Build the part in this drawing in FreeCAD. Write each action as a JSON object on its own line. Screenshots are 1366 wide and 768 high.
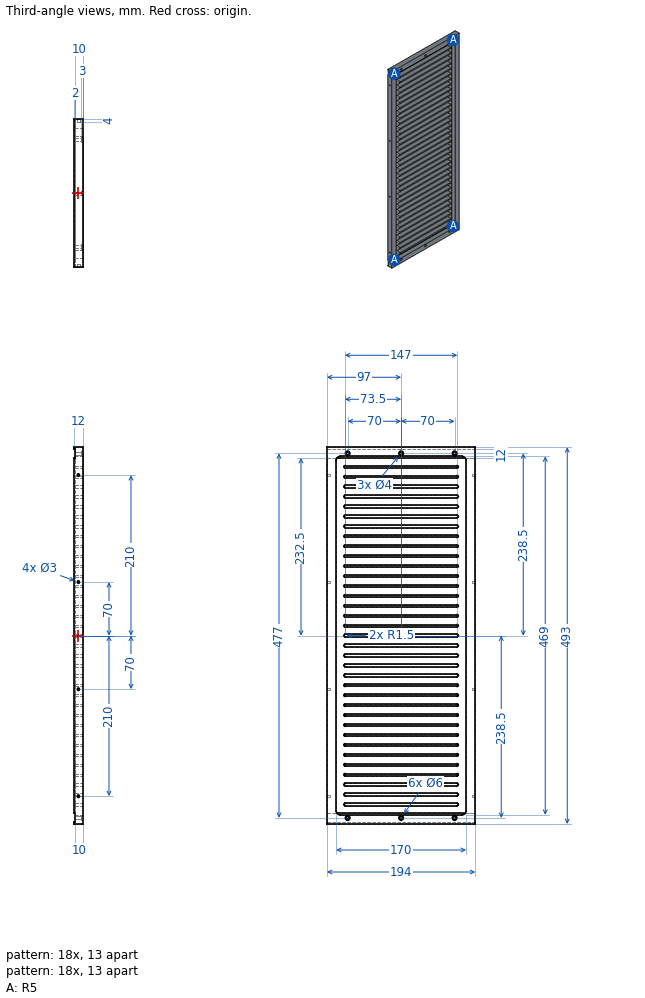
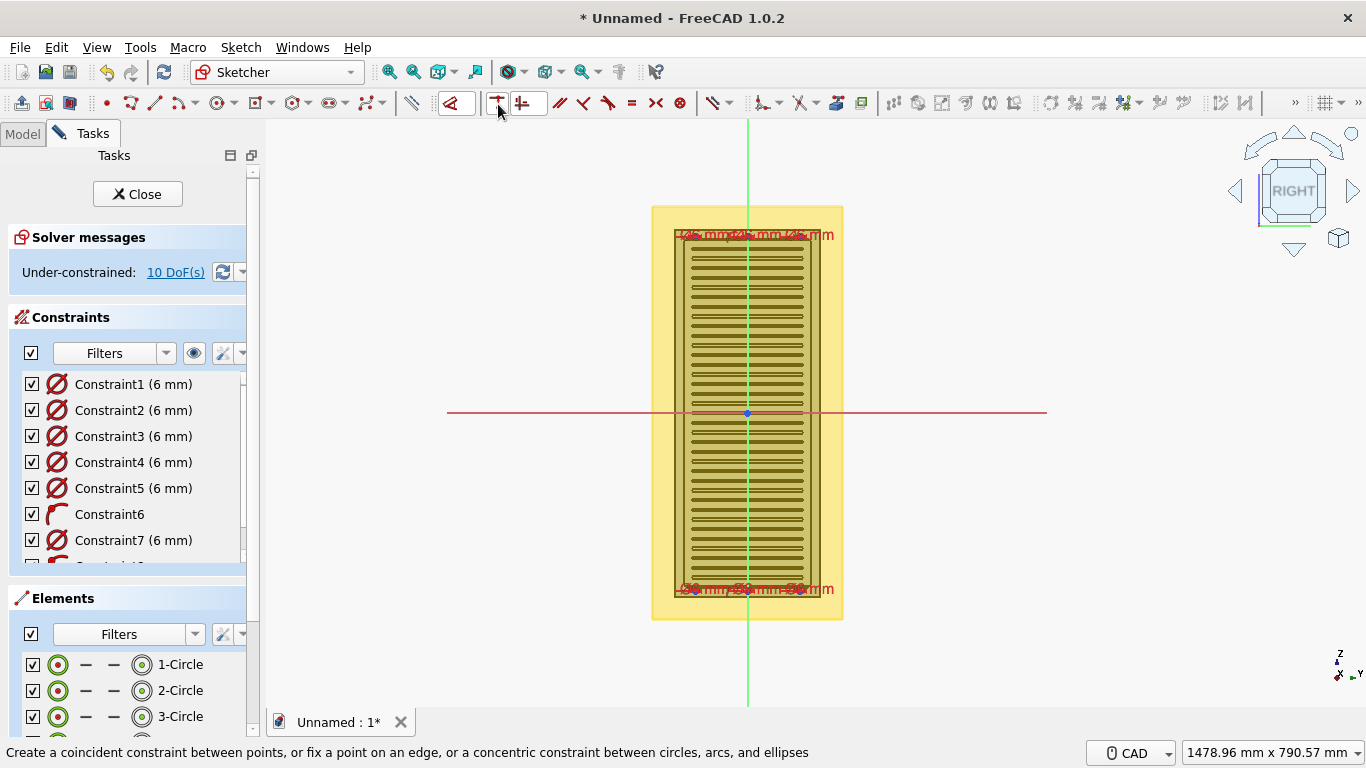
{"action": "left_click", "coordinate": [748, 591]}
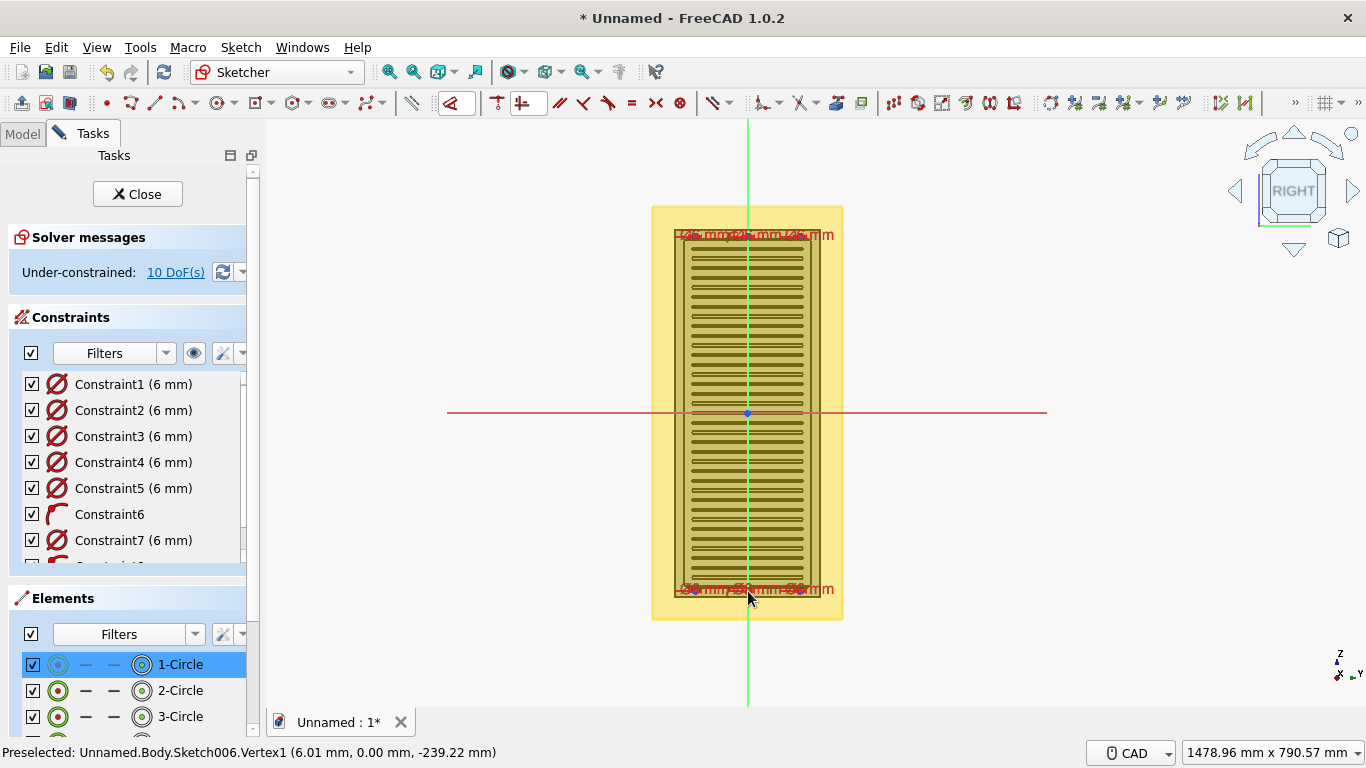
{"action": "left_click", "coordinate": [800, 591]}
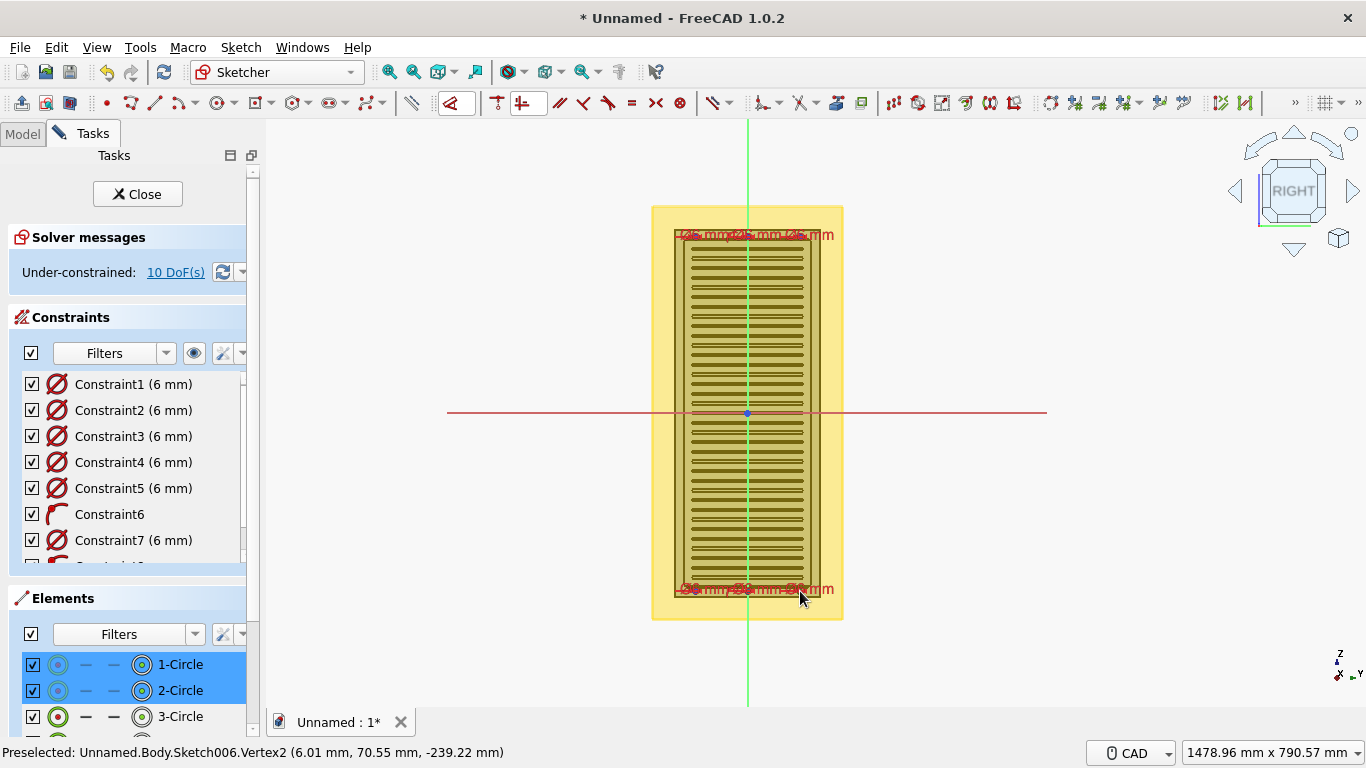
{"action": "key", "text": "h"}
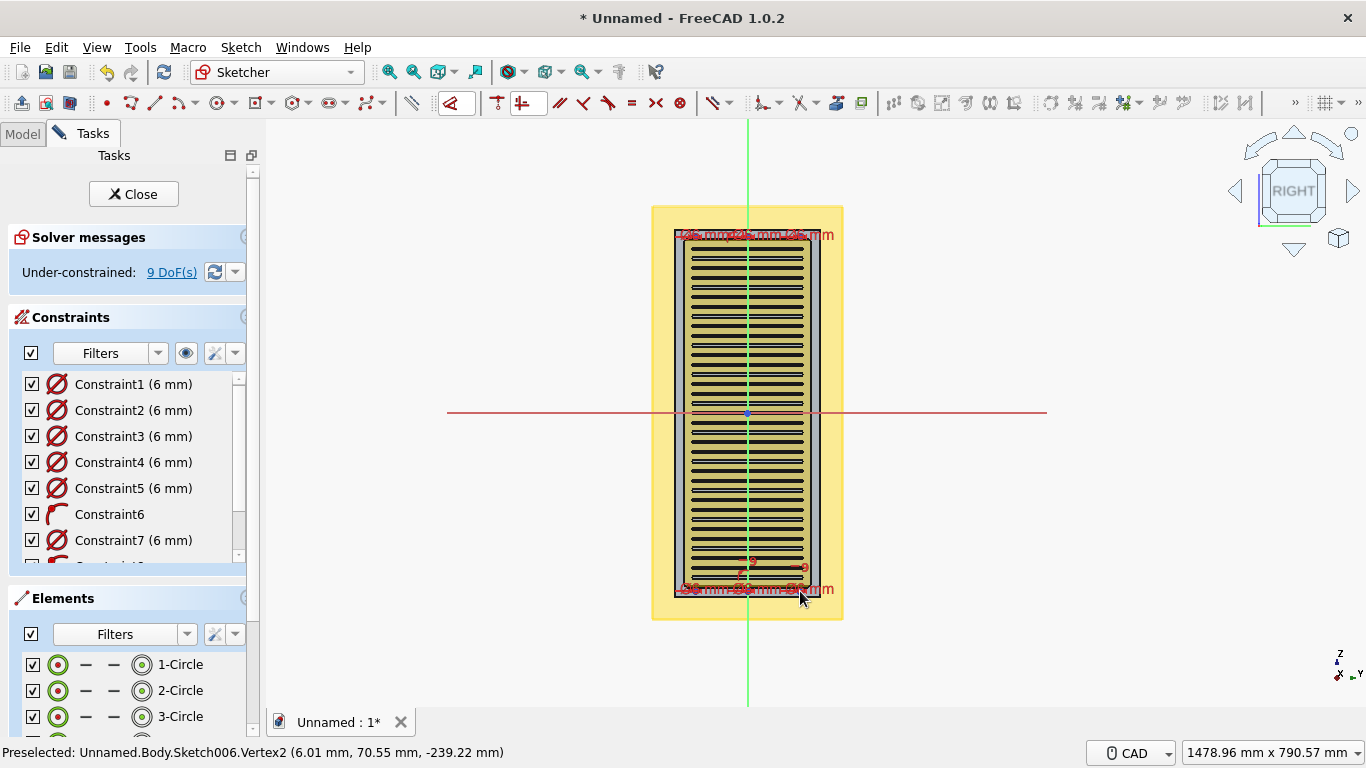
{"action": "left_click", "coordinate": [748, 591]}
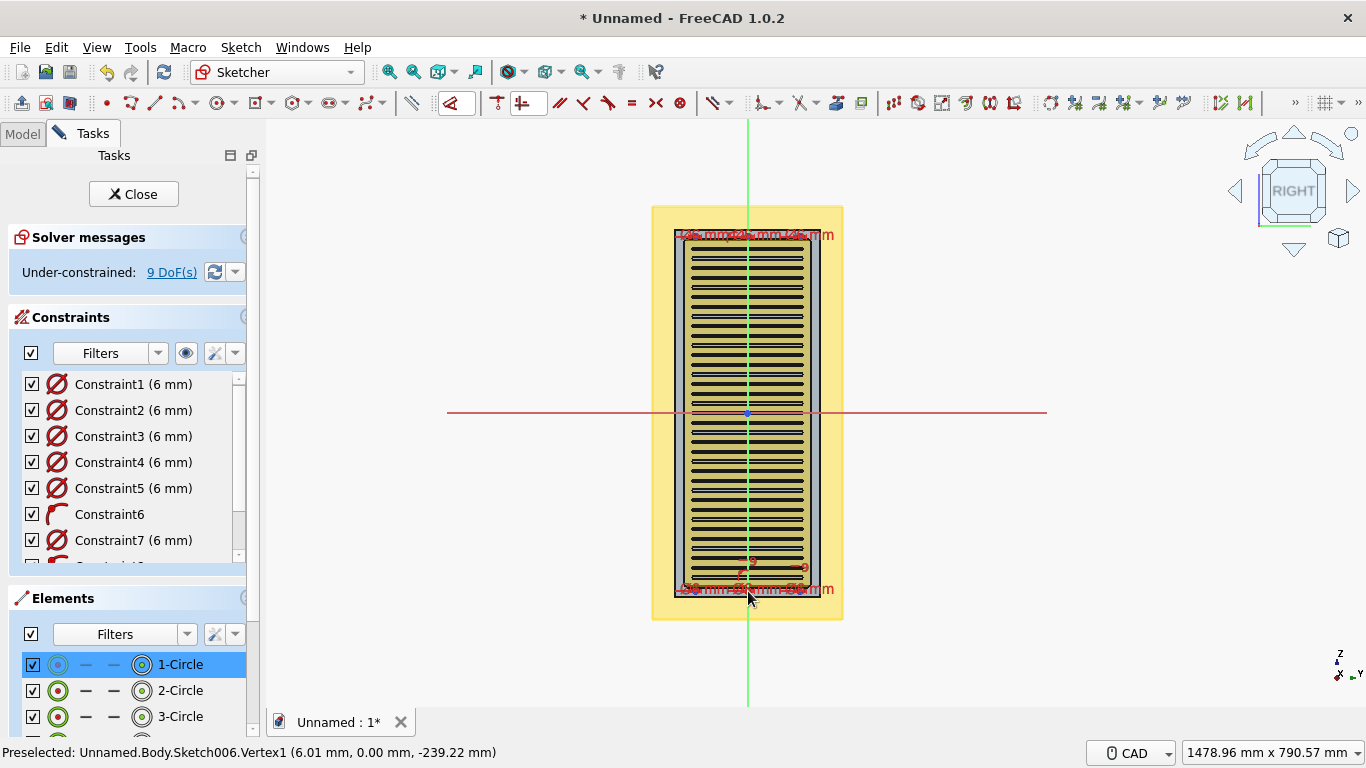
{"action": "left_click", "coordinate": [695, 591]}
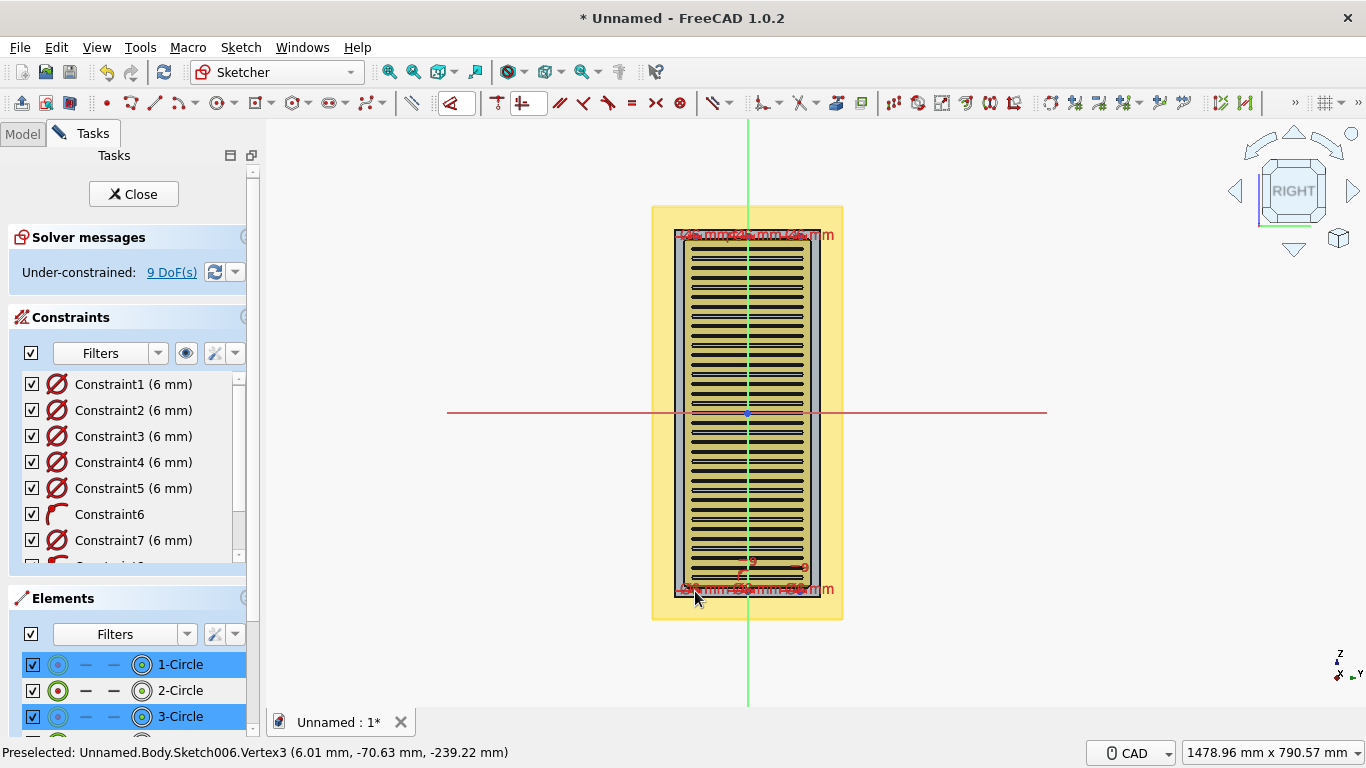
{"action": "key", "text": "h"}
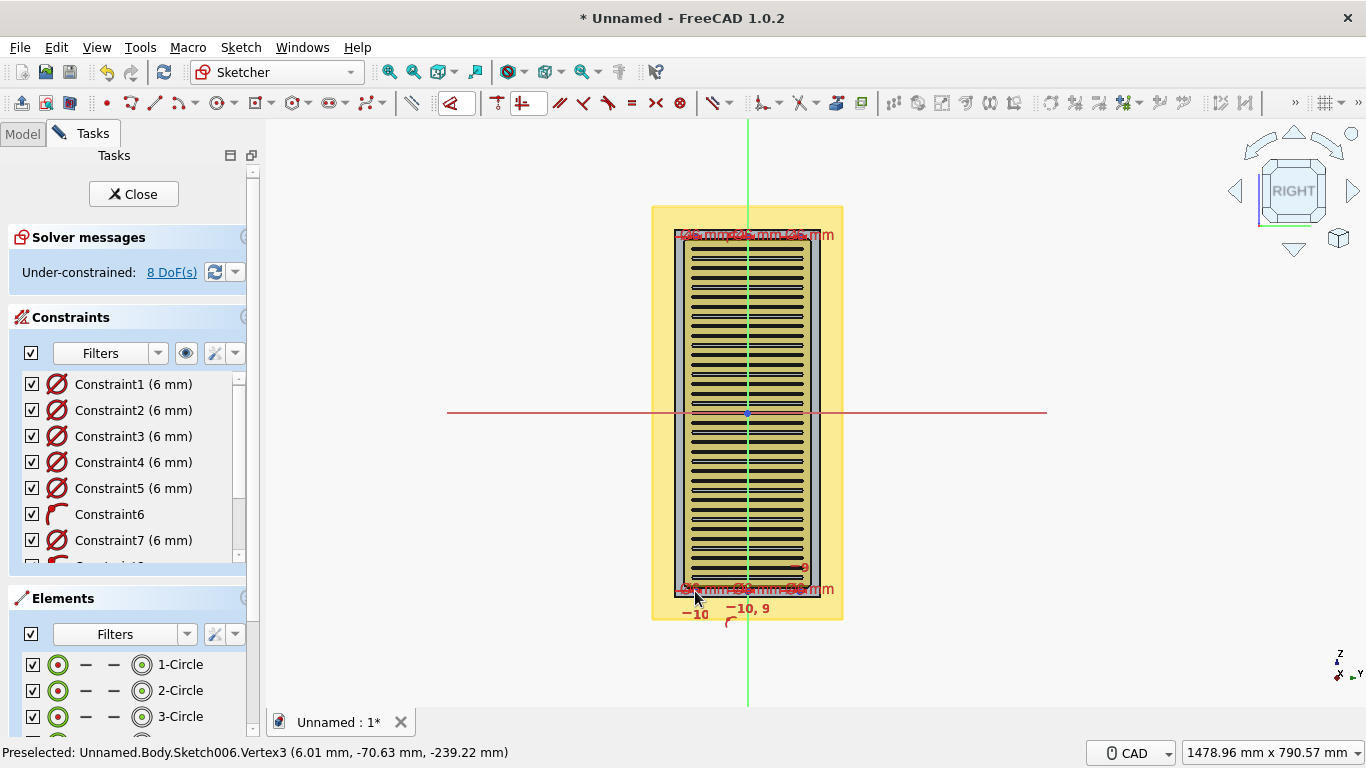
{"action": "left_click", "coordinate": [695, 591]}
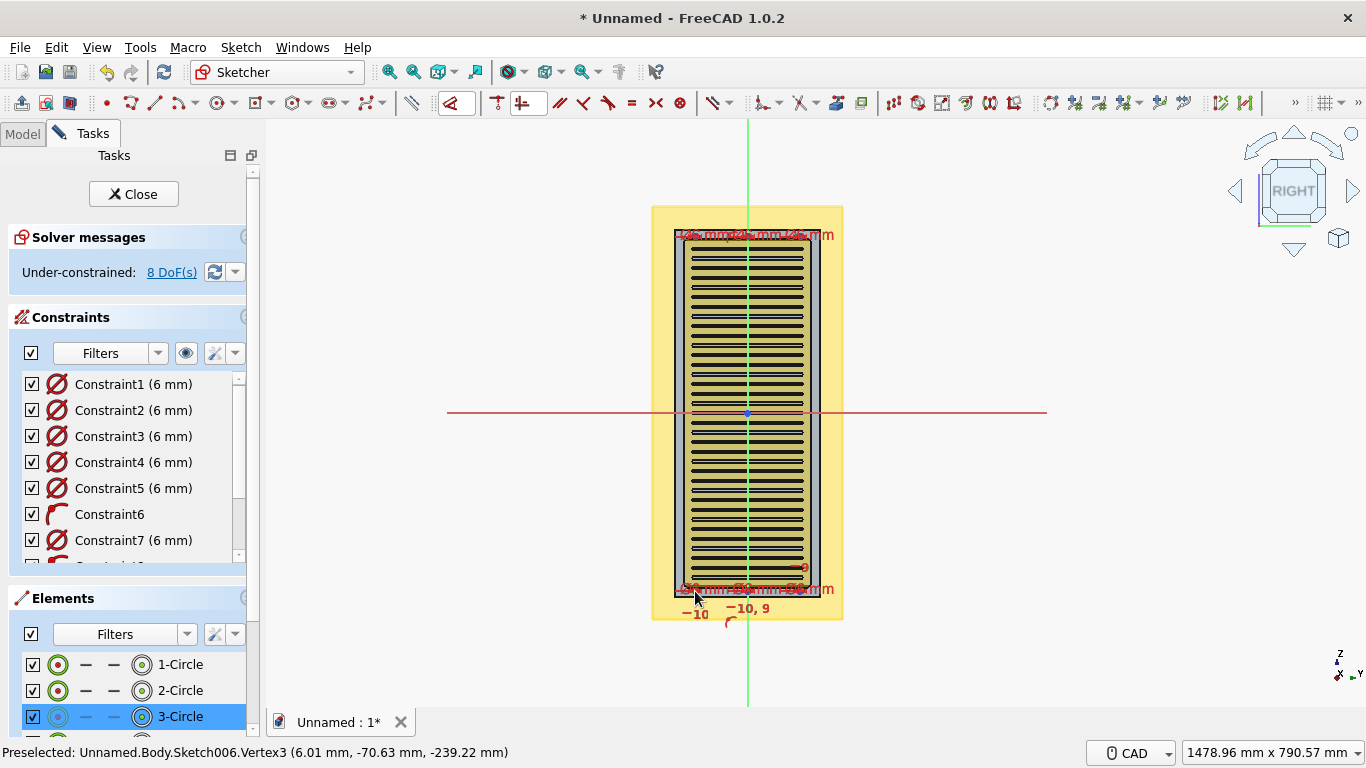
{"action": "left_click", "coordinate": [695, 237]}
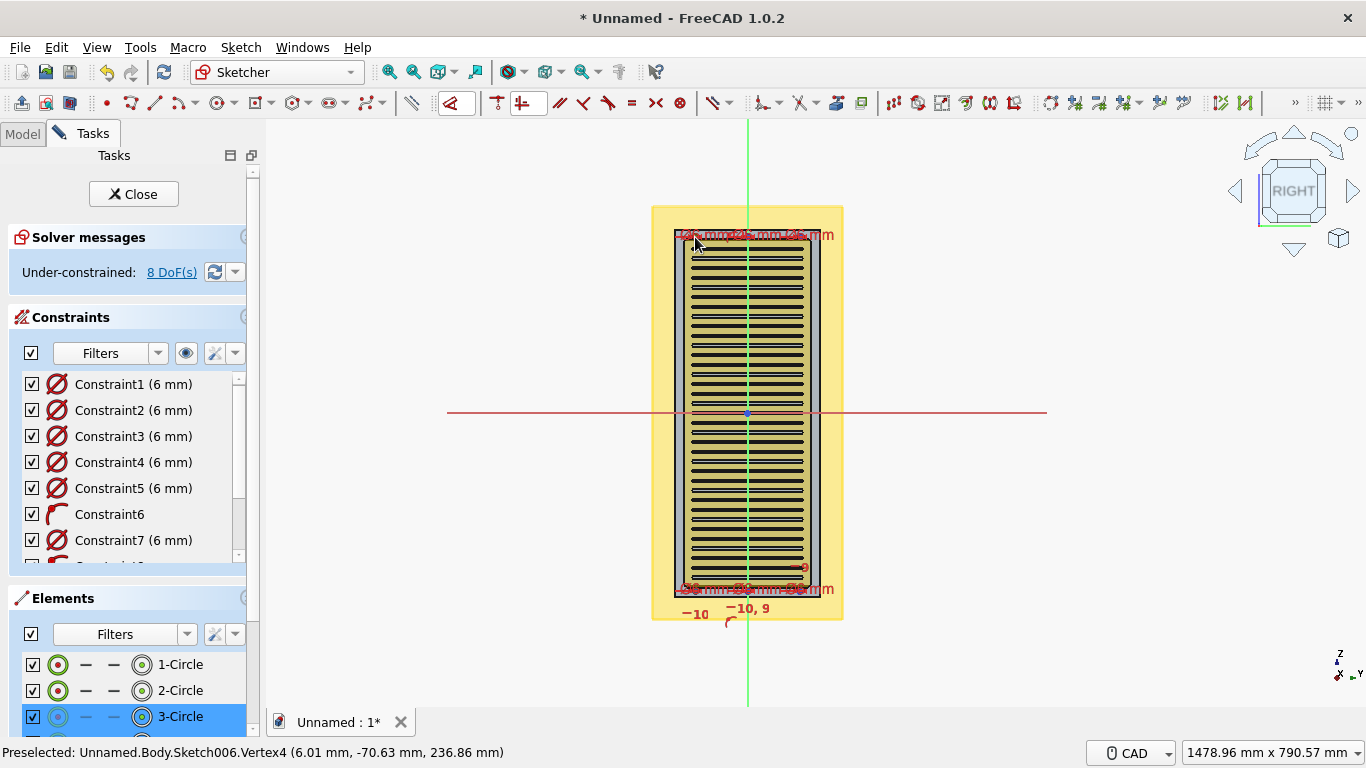
{"action": "left_click", "coordinate": [542, 104]}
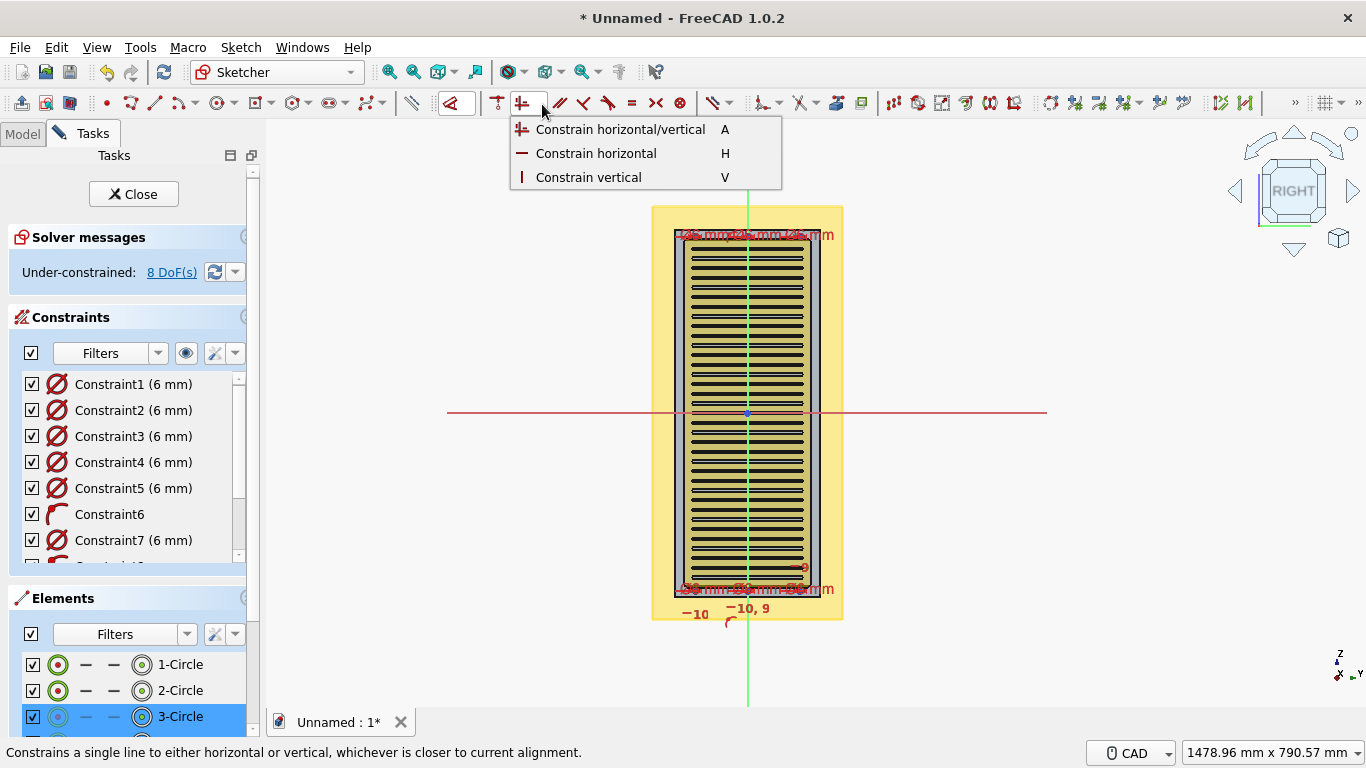
{"action": "left_click", "coordinate": [646, 177]}